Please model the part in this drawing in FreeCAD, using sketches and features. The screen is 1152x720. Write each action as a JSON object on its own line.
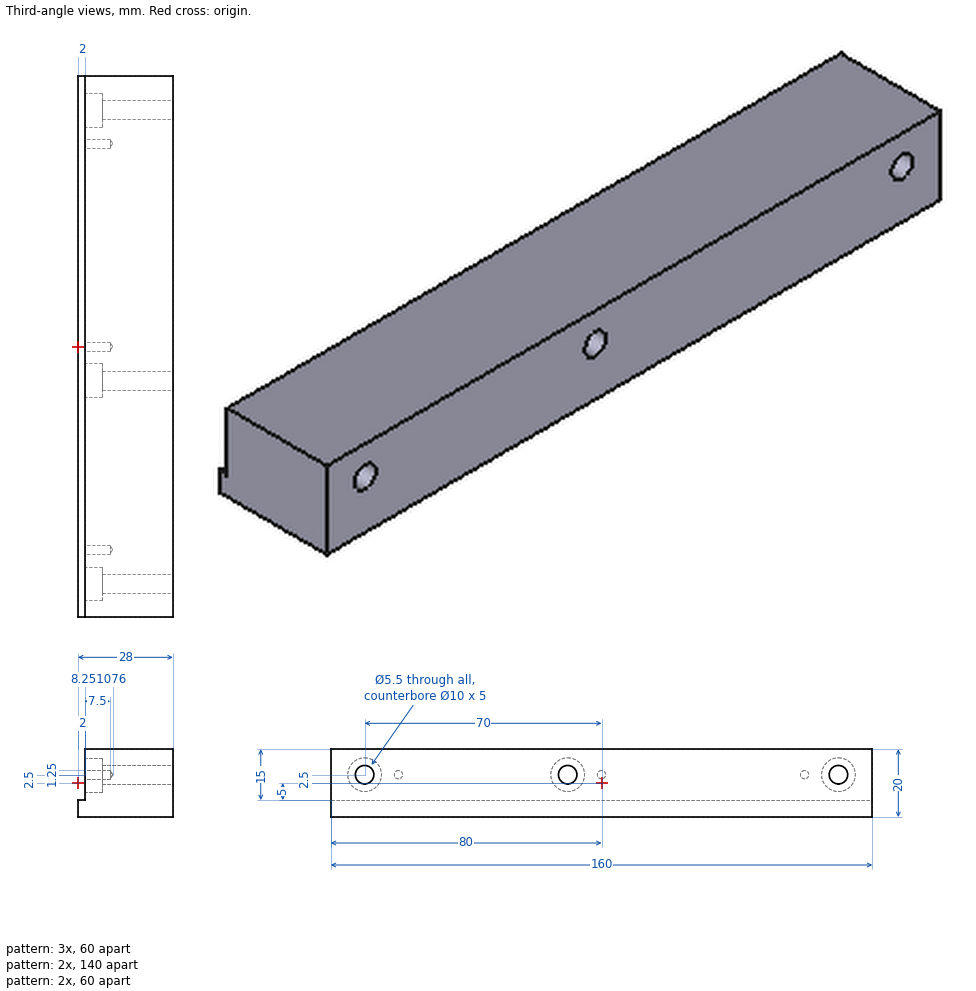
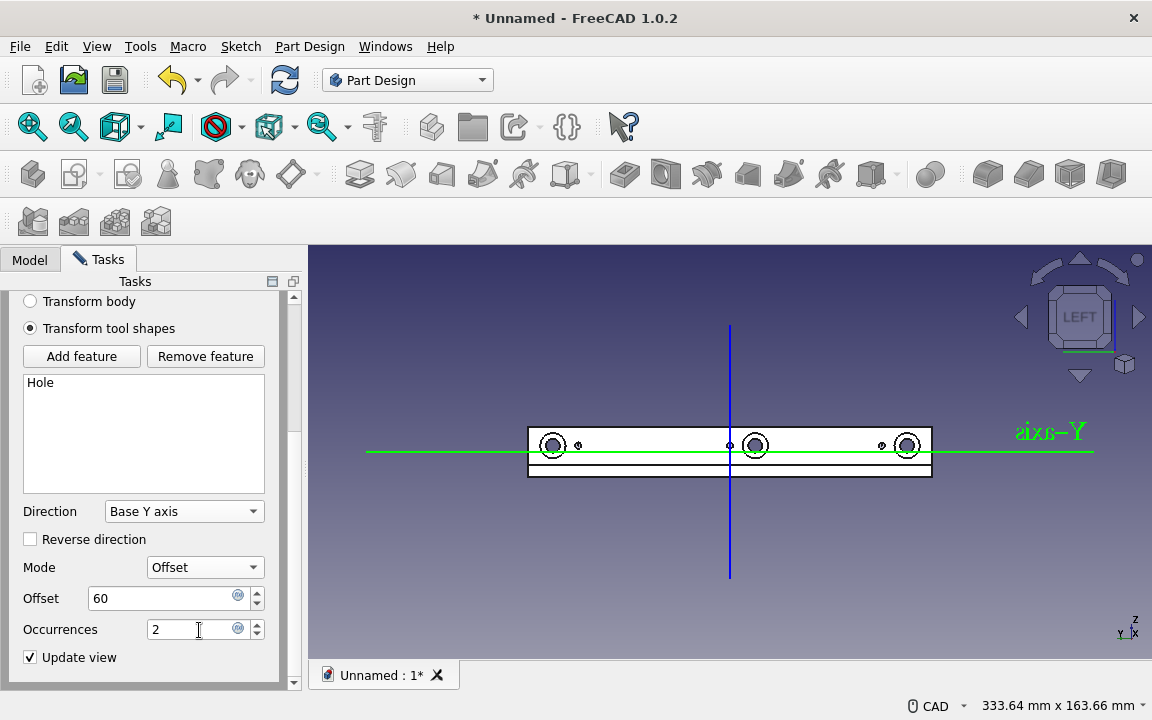
{"action": "type", "text": "2"}
{"action": "key", "text": "Tab"}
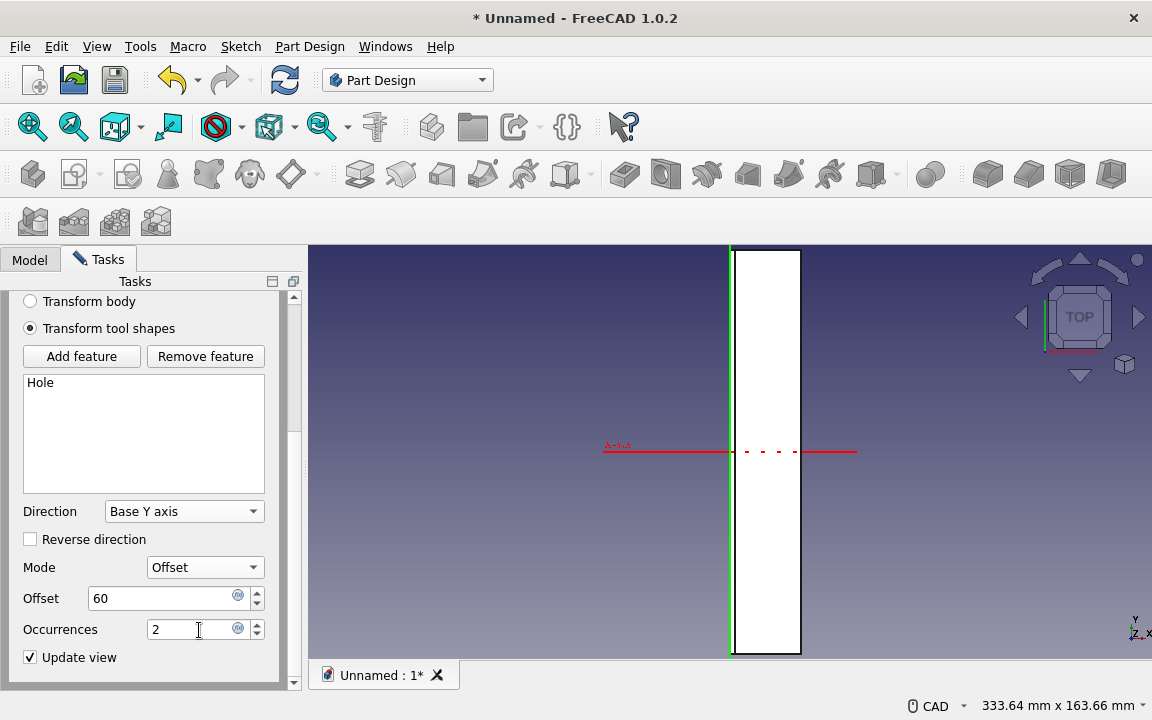
{"action": "scroll", "coordinate": [294, 490], "scroll_direction": "up", "scroll_amount": 5}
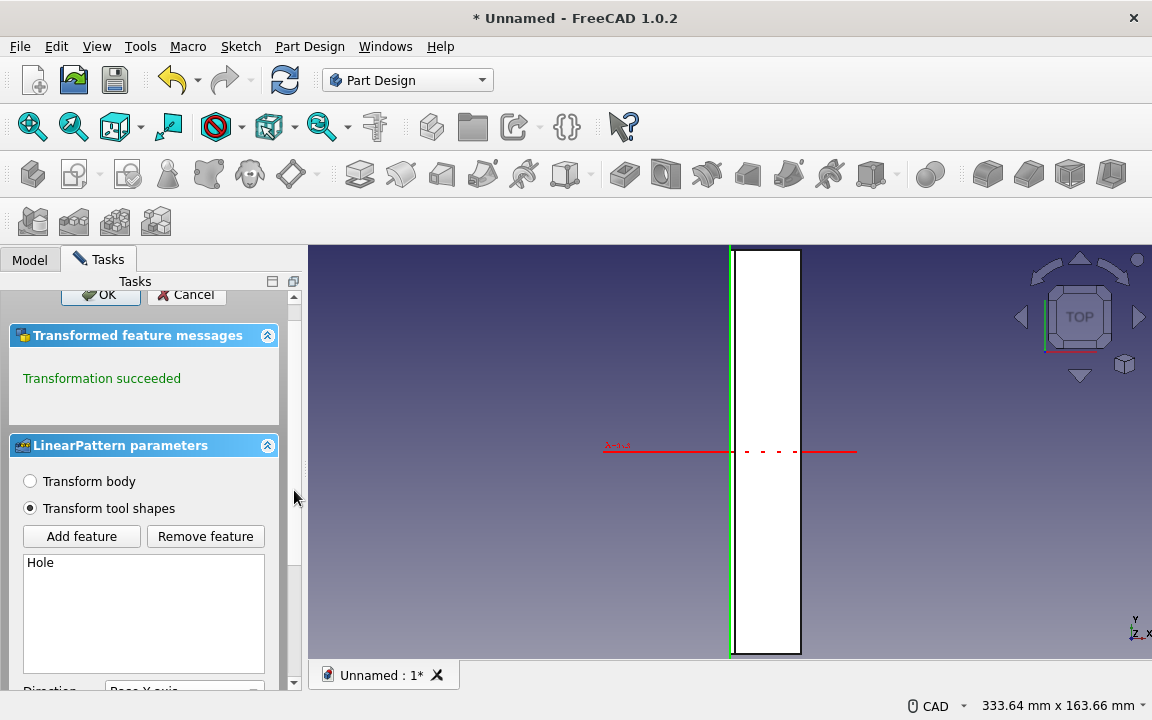
{"action": "left_click", "coordinate": [101, 320]}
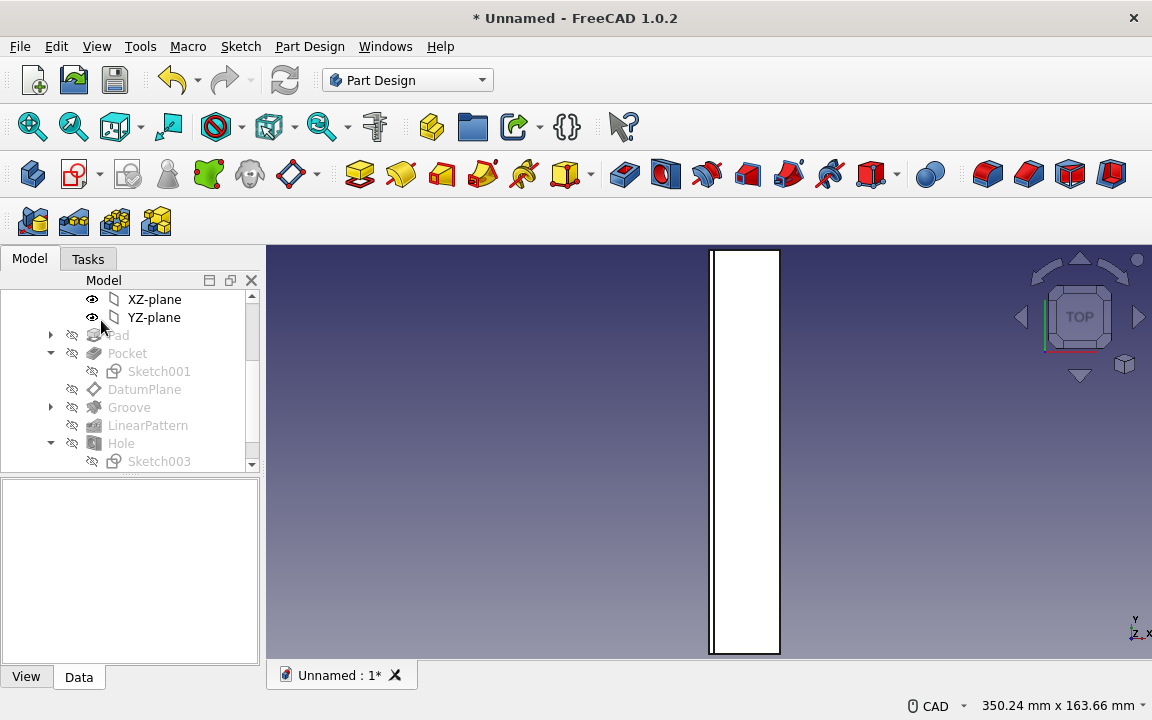
{"action": "key", "text": "0"}